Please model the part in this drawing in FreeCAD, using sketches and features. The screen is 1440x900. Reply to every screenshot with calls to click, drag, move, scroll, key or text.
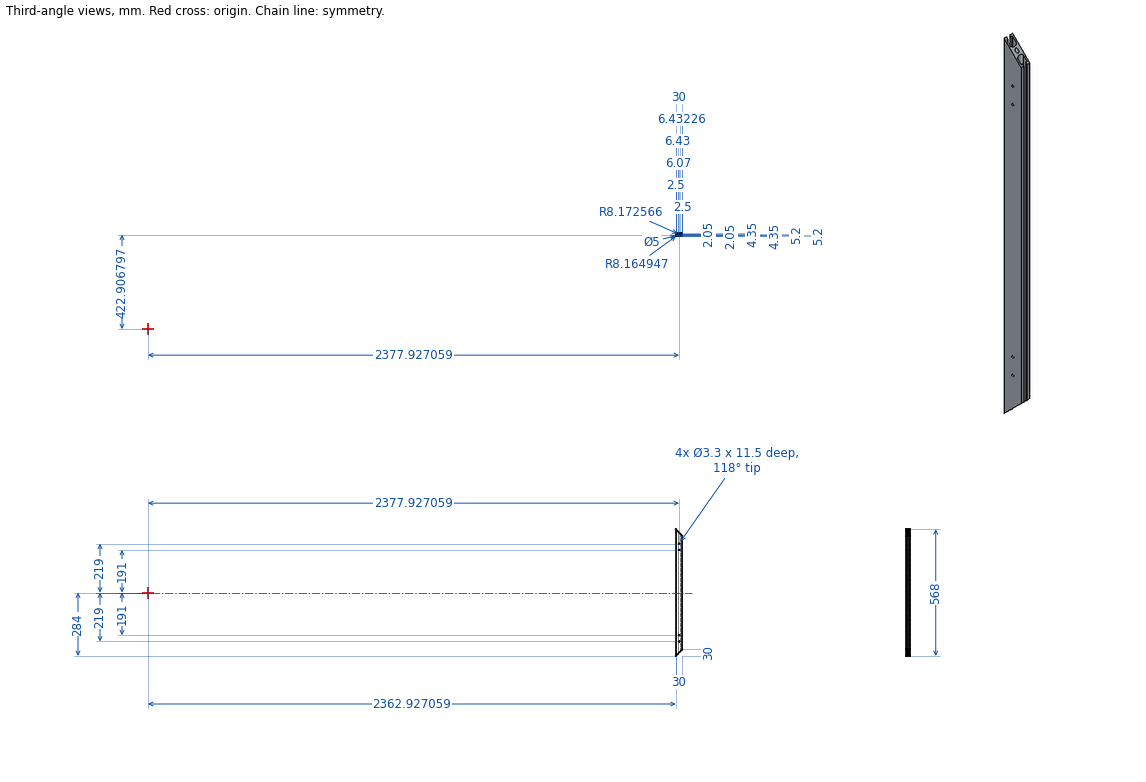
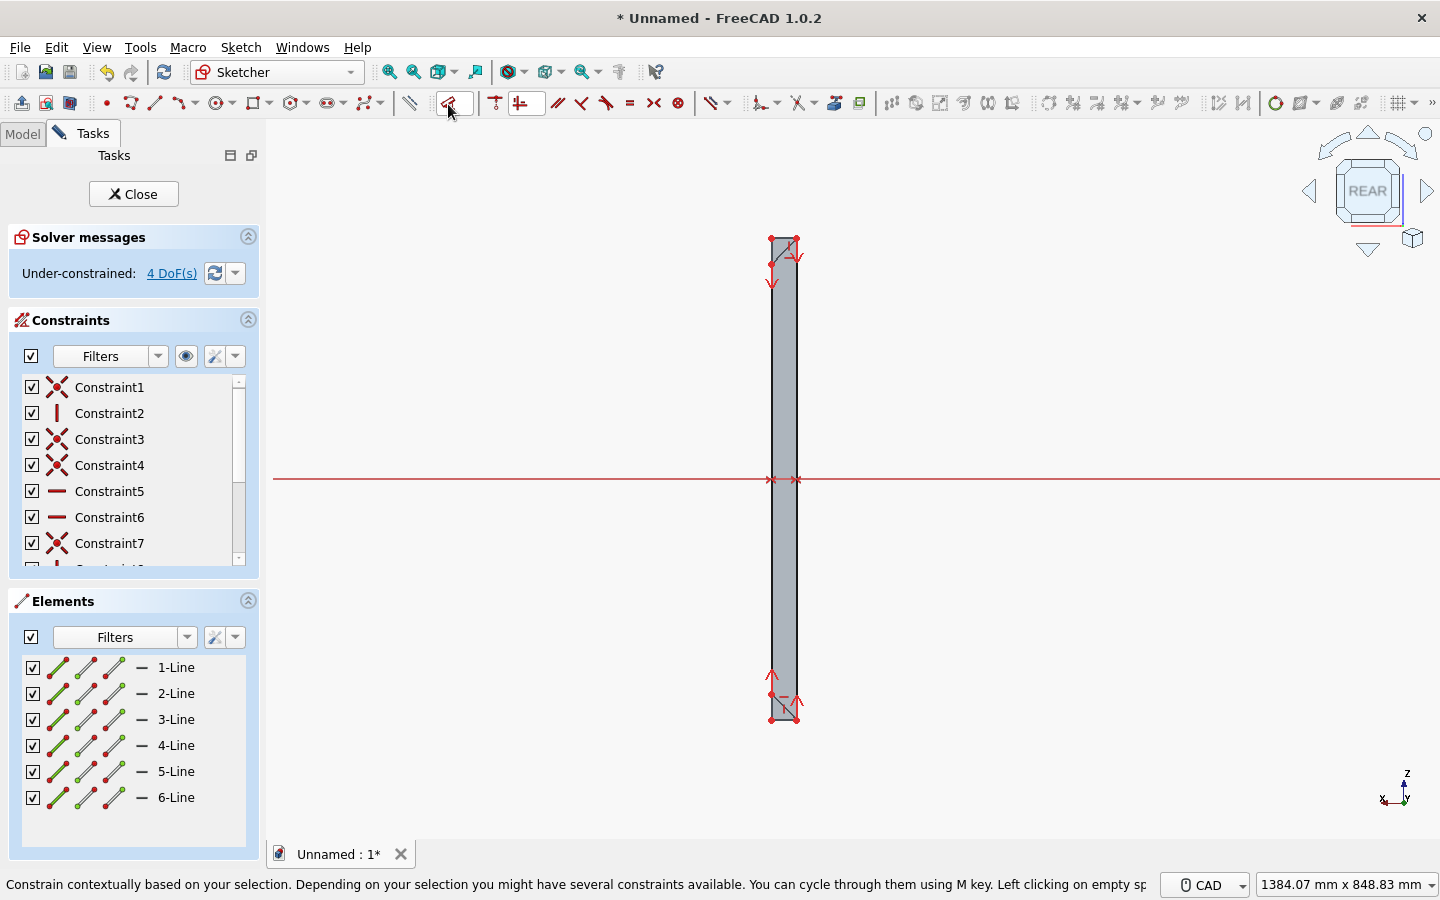
scroll(772, 710, up, 3)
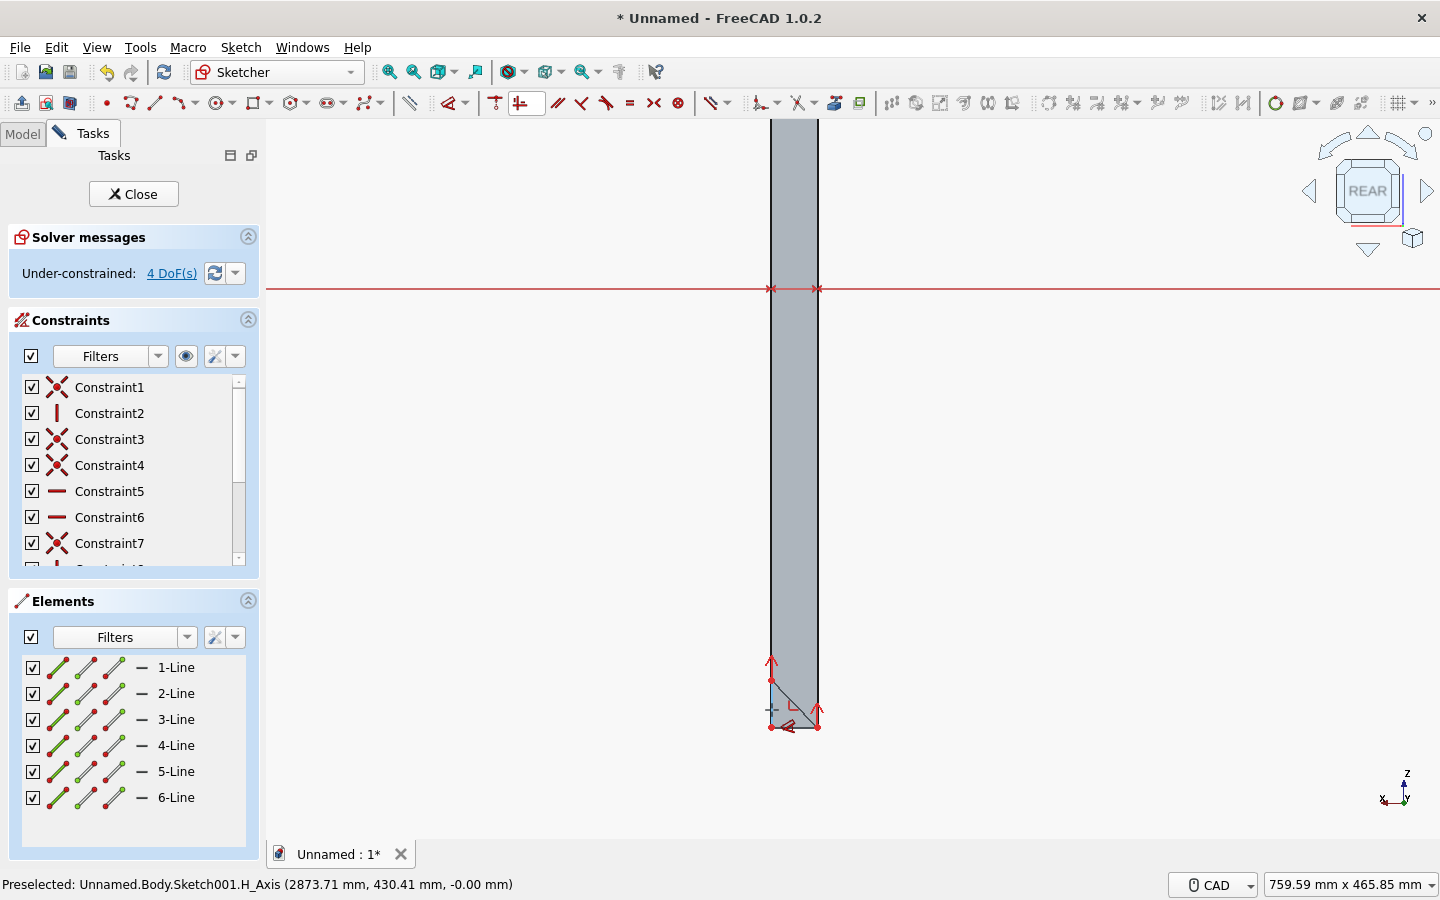
click(772, 709)
click(738, 704)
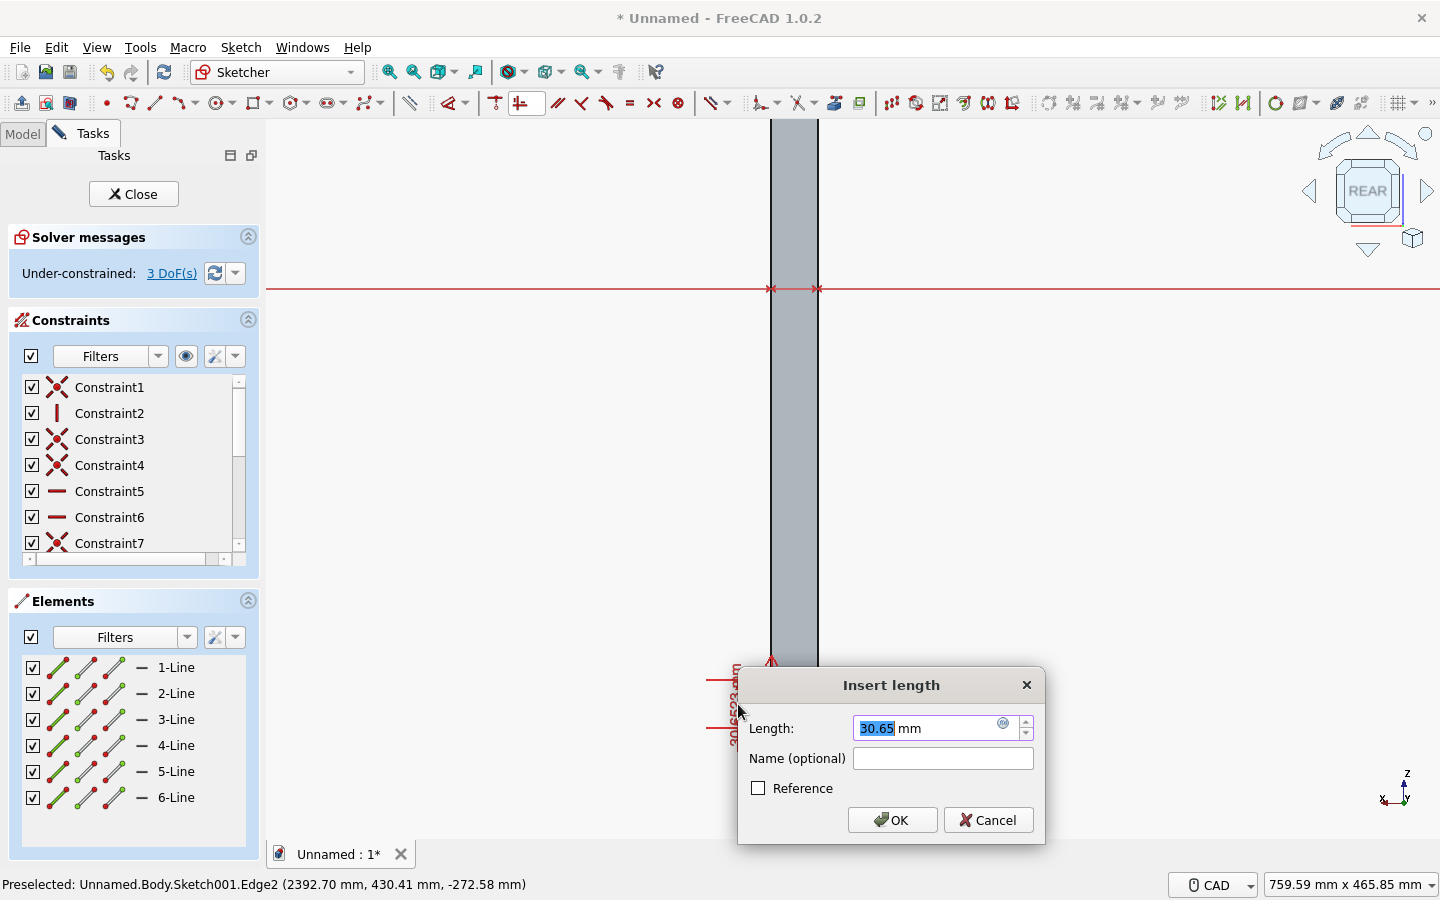
text(30)
key(Return)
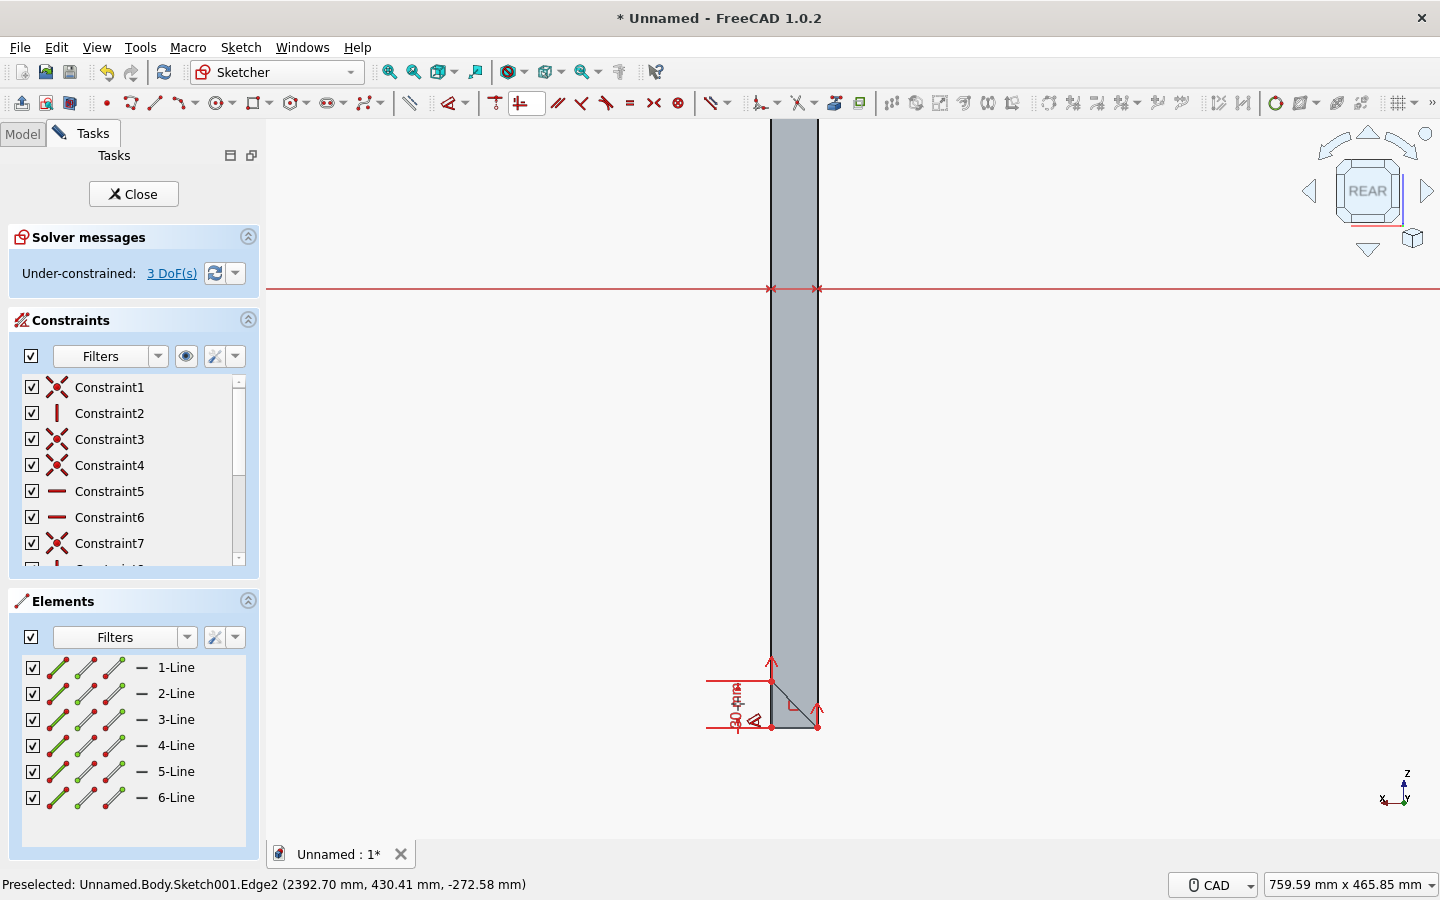
click(785, 728)
click(794, 762)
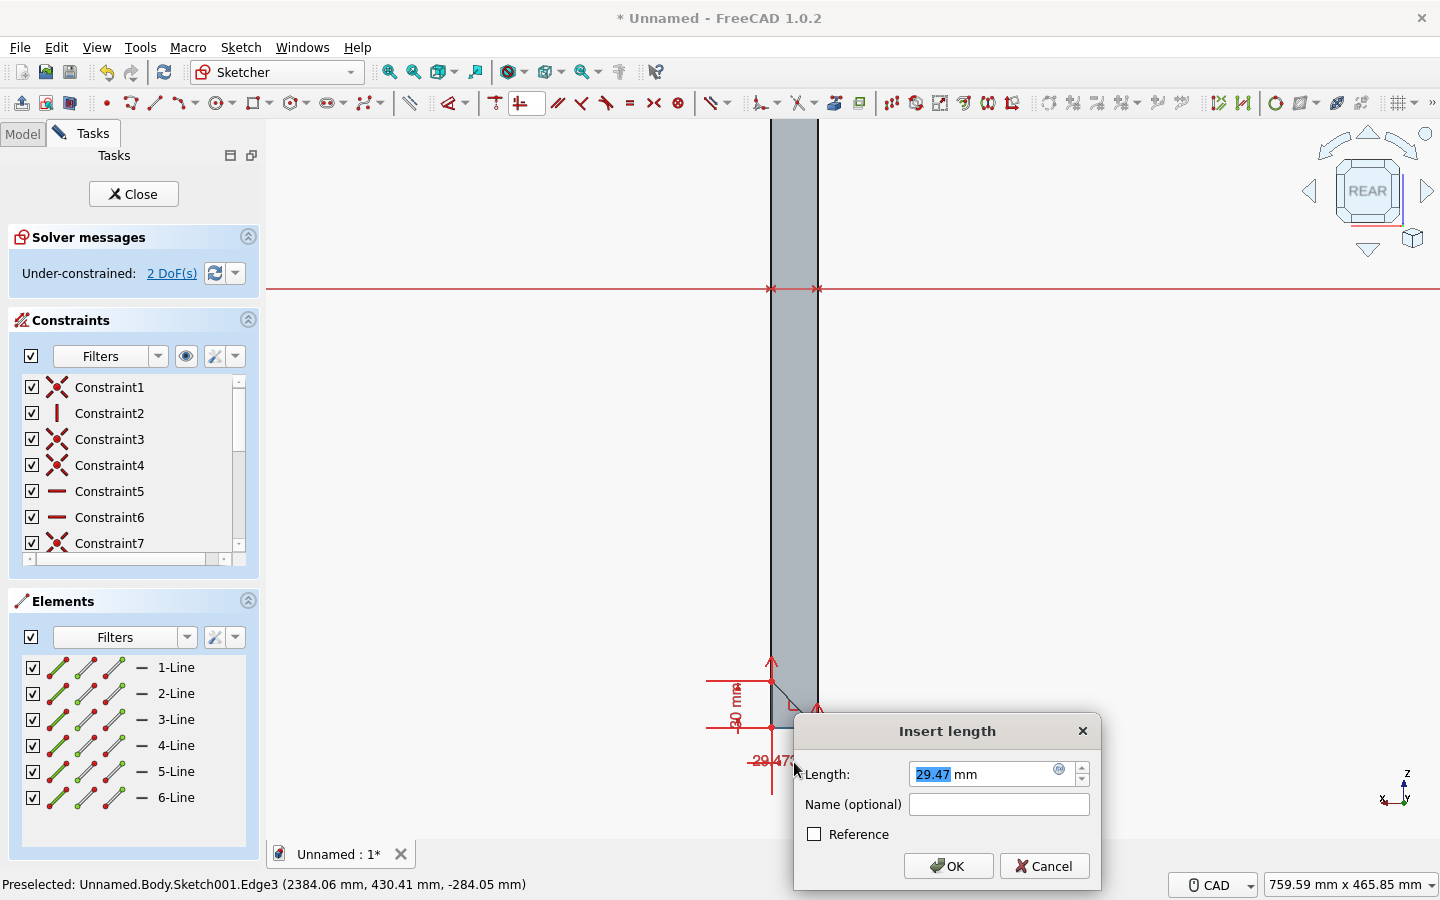
text(30)
key(Return)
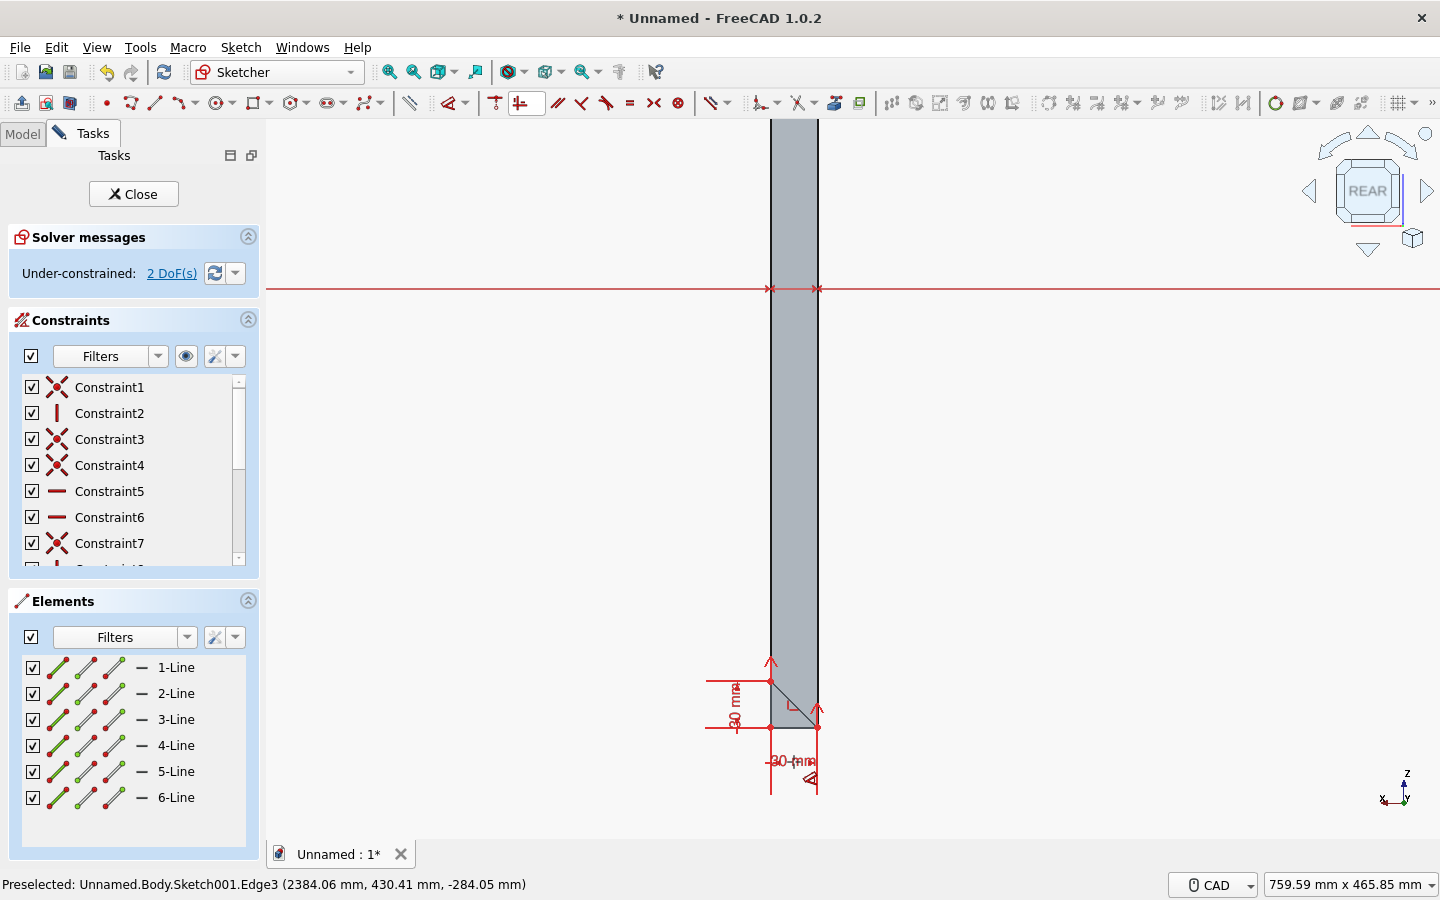
click(817, 728)
click(783, 508)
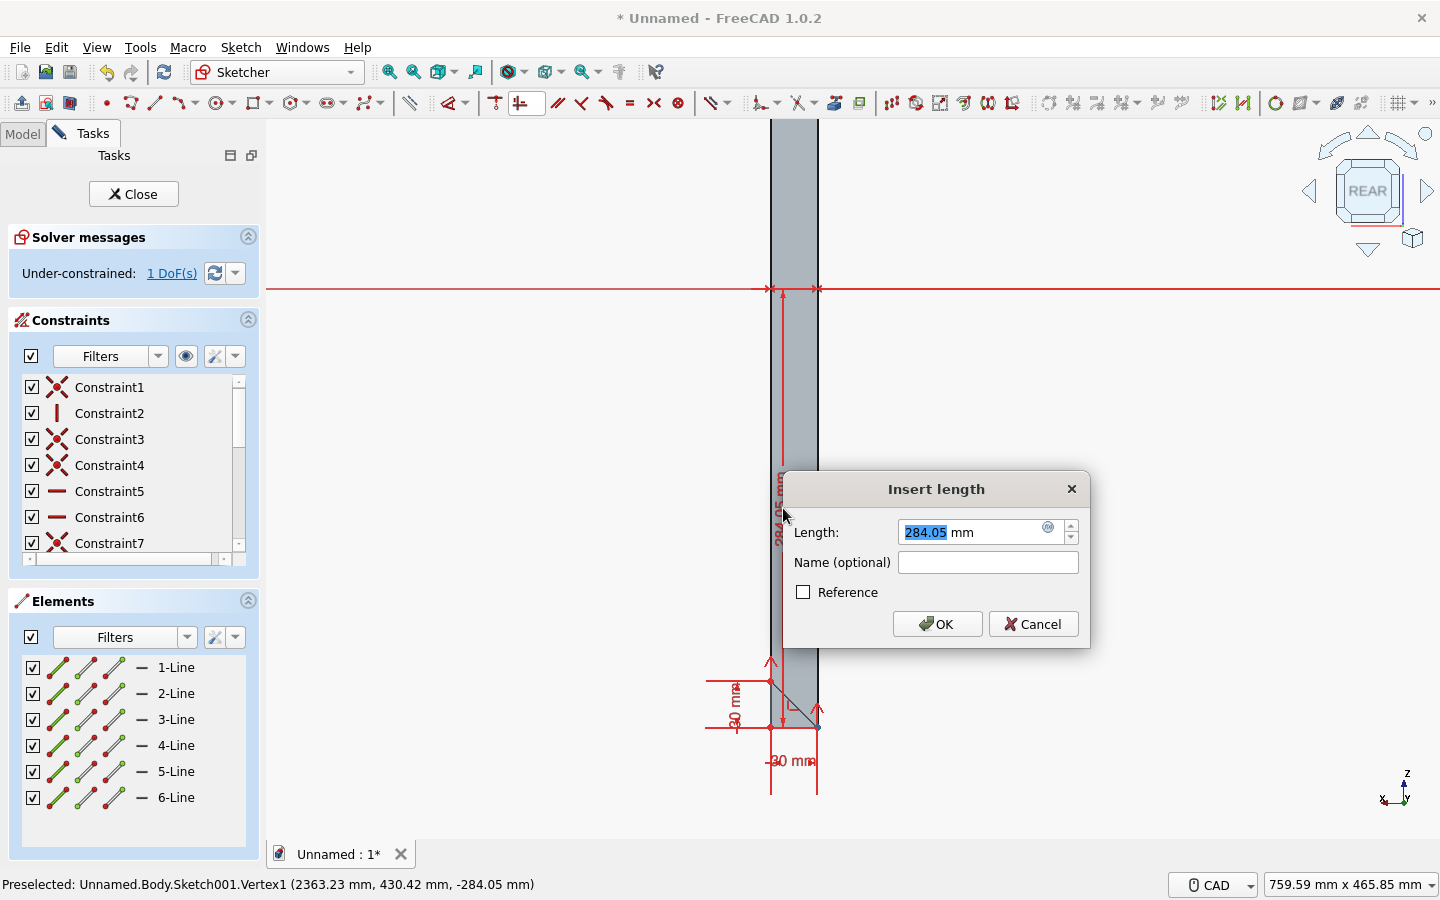
text(284)
key(Return)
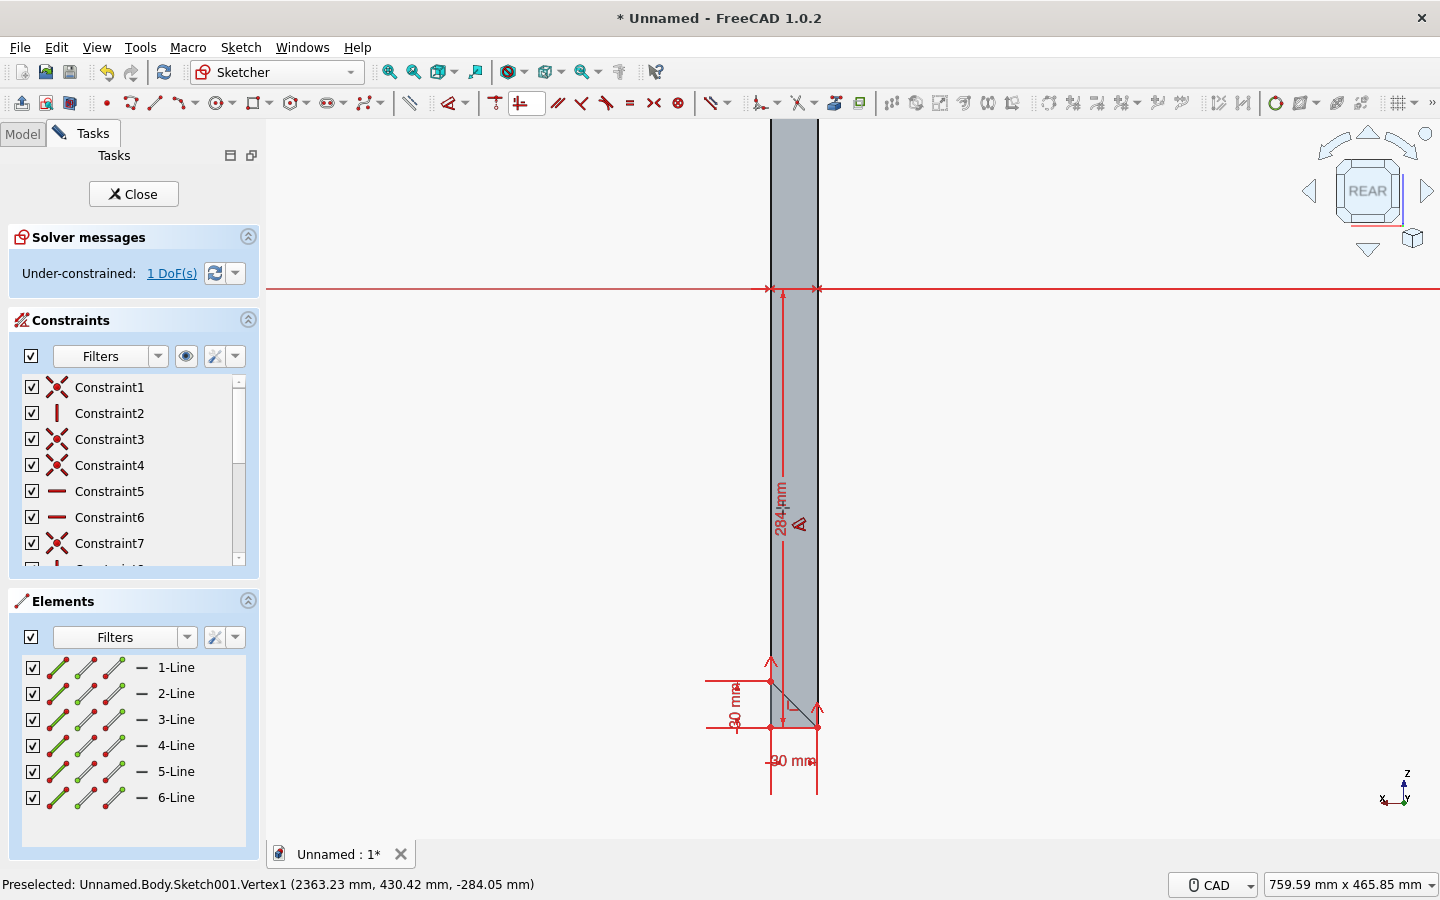
click(817, 728)
click(1046, 762)